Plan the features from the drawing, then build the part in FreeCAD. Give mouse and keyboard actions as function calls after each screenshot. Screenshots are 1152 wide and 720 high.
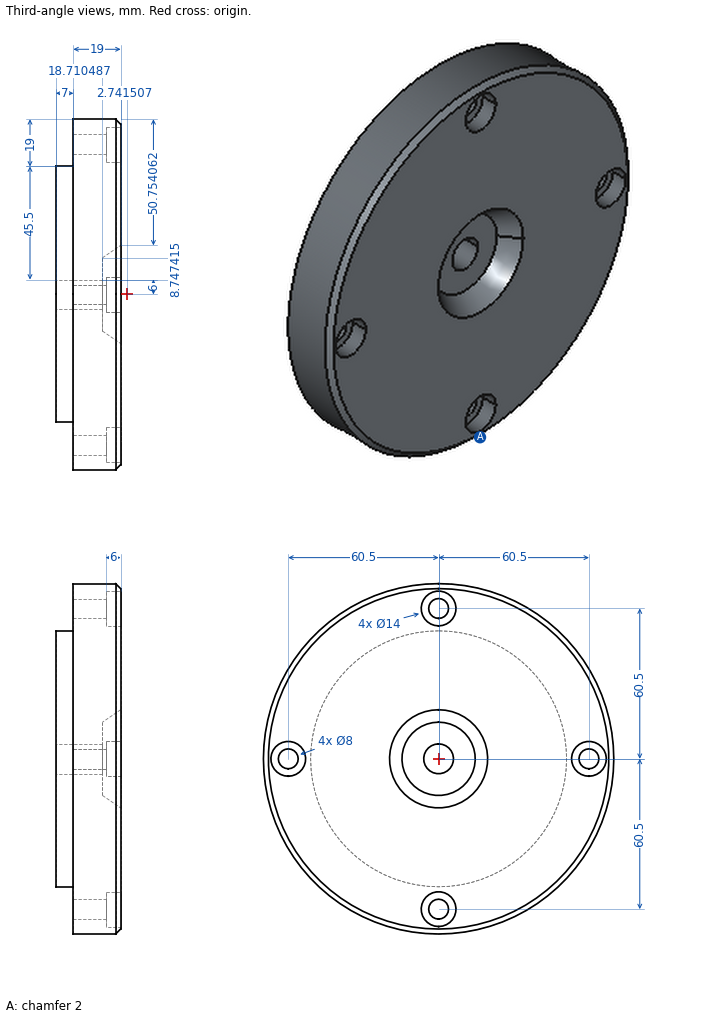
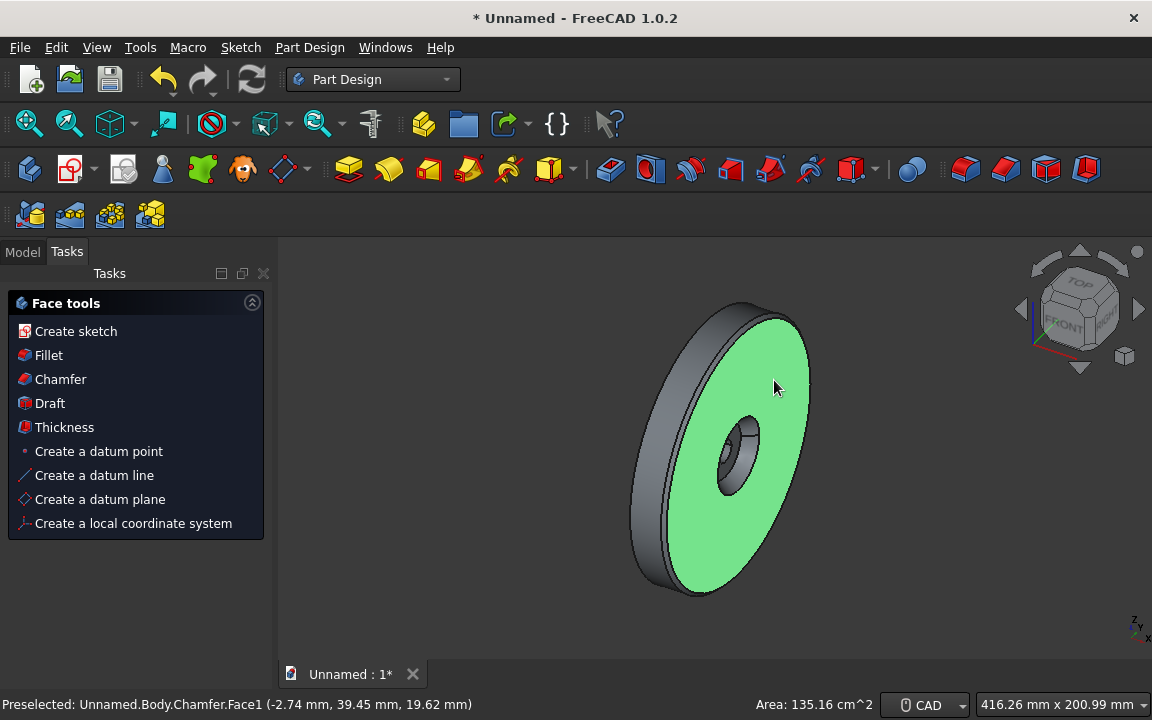
click(70, 170)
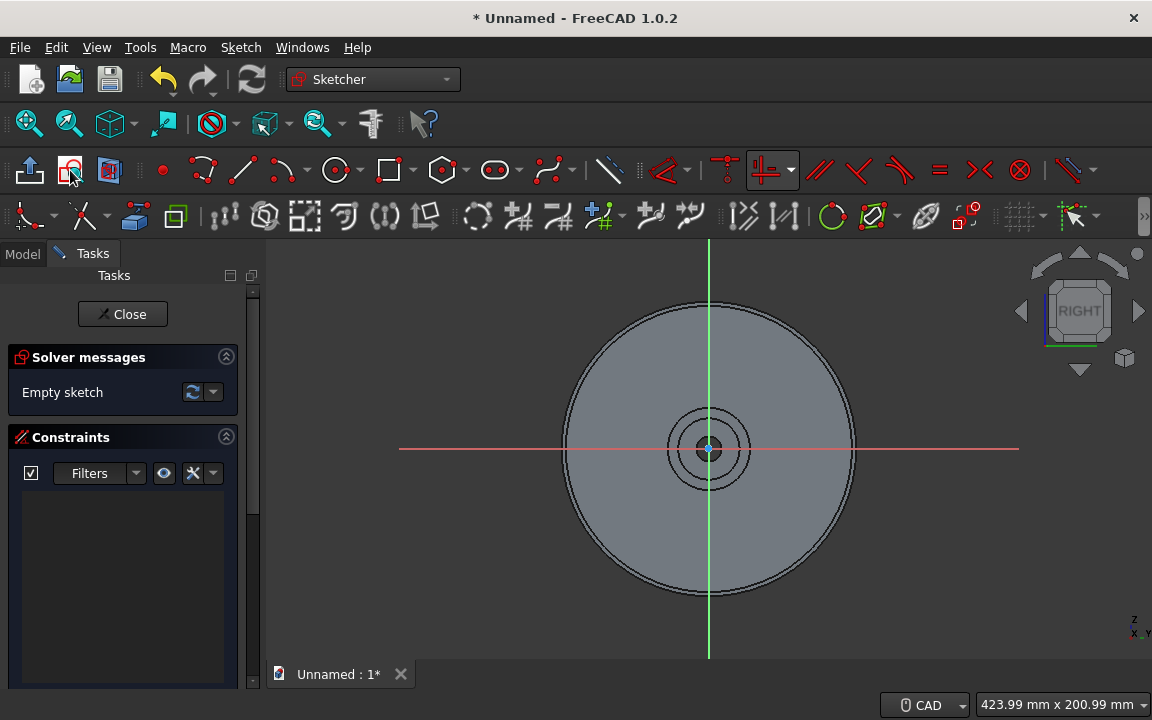
key(g)
key(c)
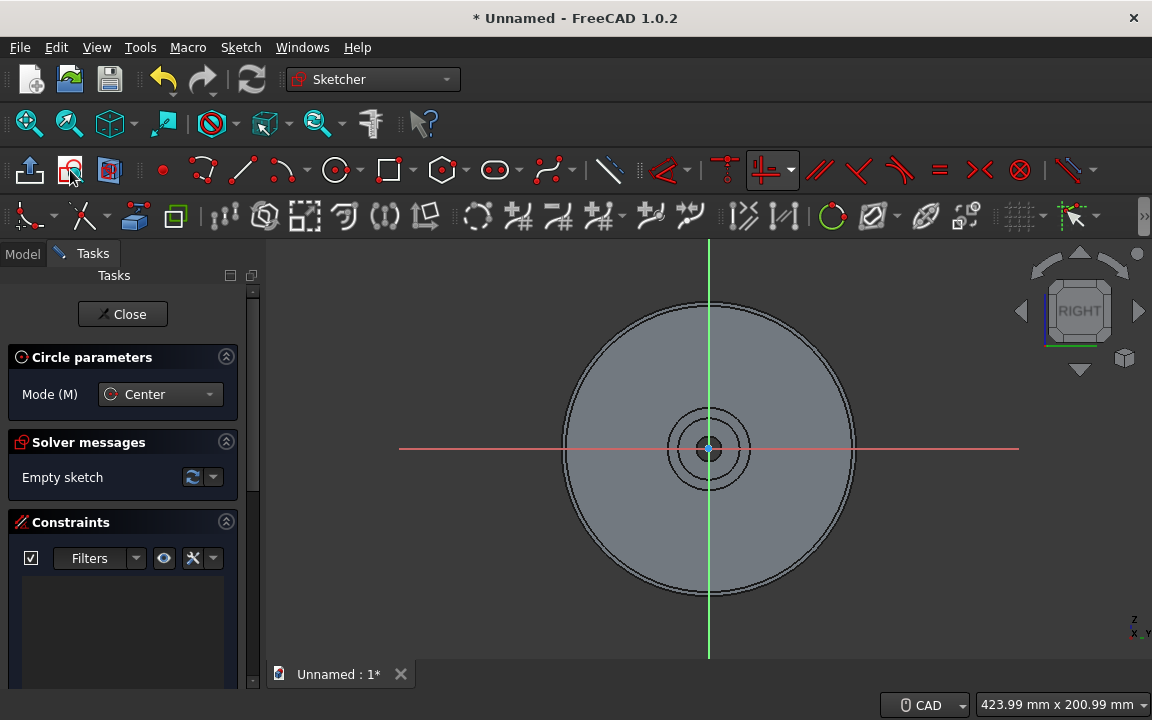
scroll(582, 449, up, 5)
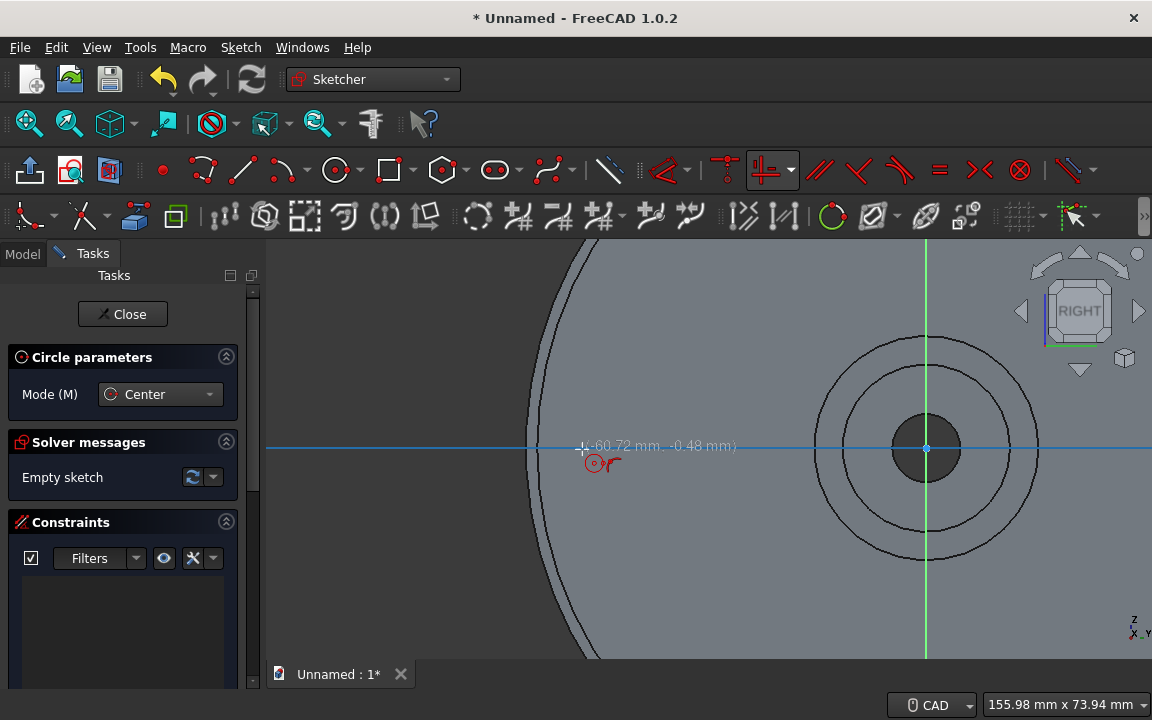
click(583, 448)
move(599, 432)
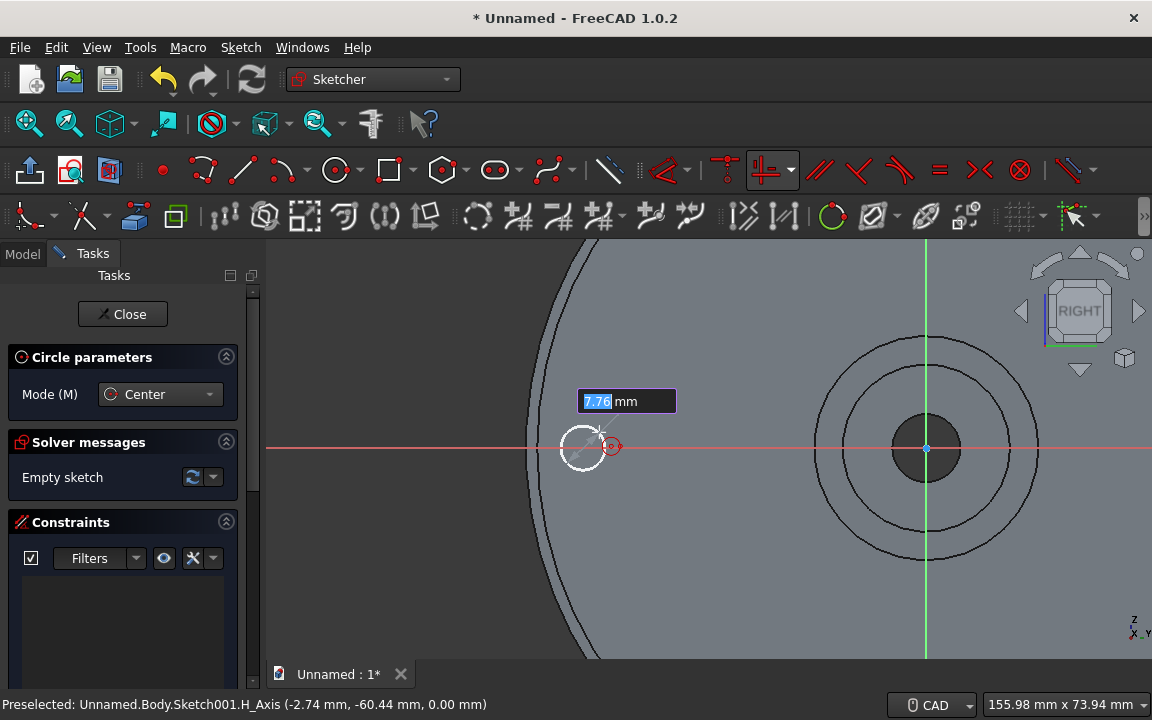
text(8)
key(Return)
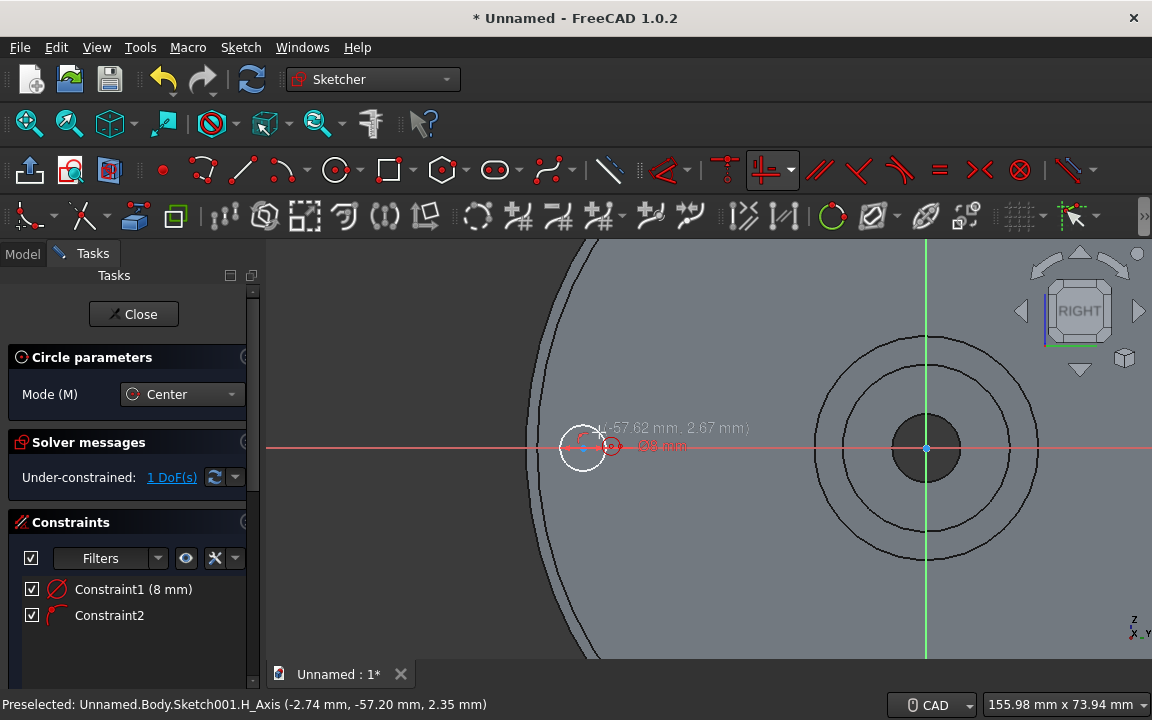
scroll(474, 450, down, 5)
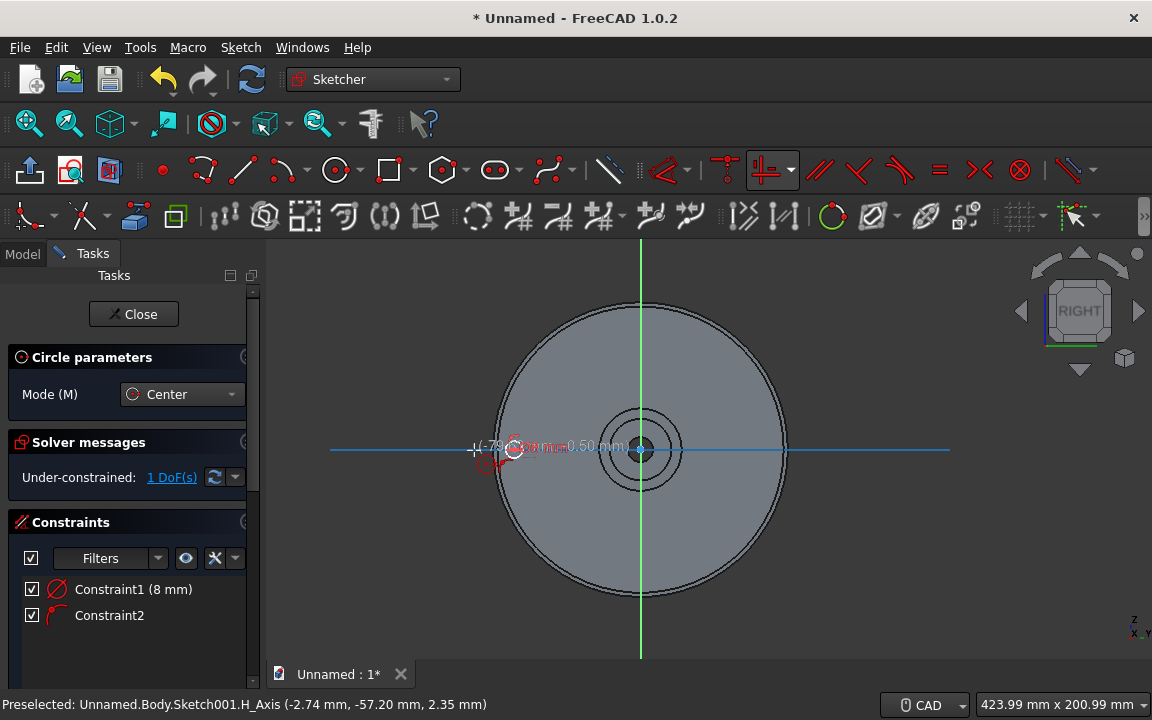
scroll(641, 323, up, 5)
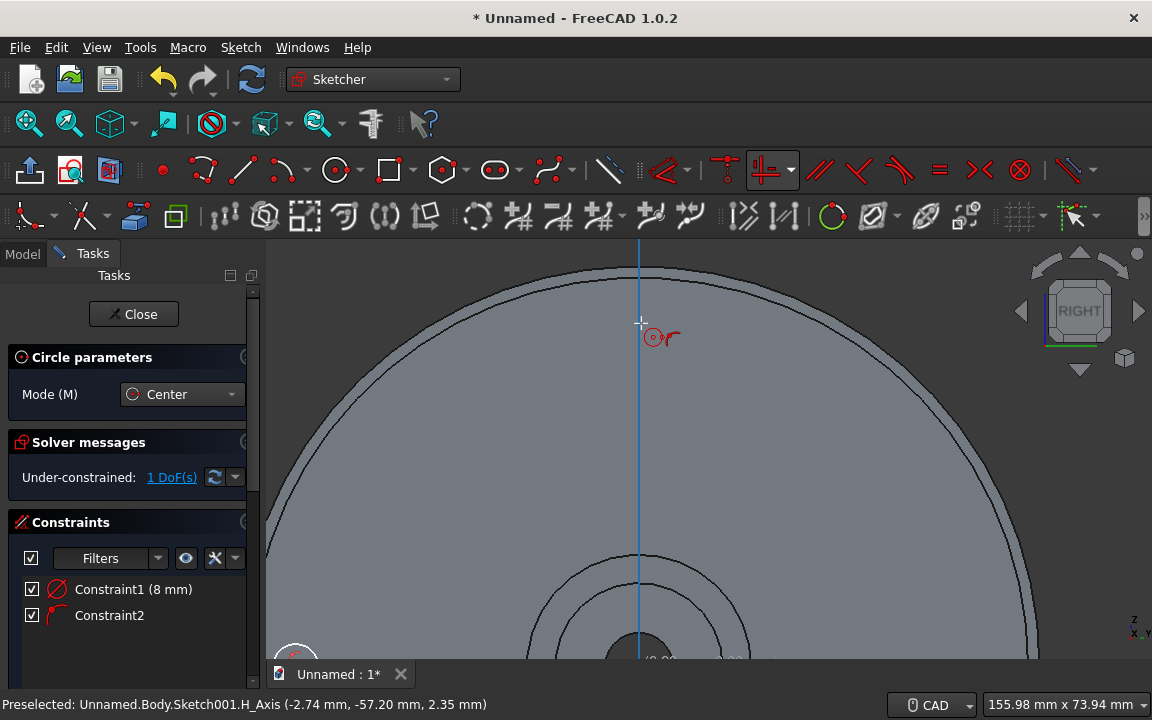
click(639, 323)
move(655, 307)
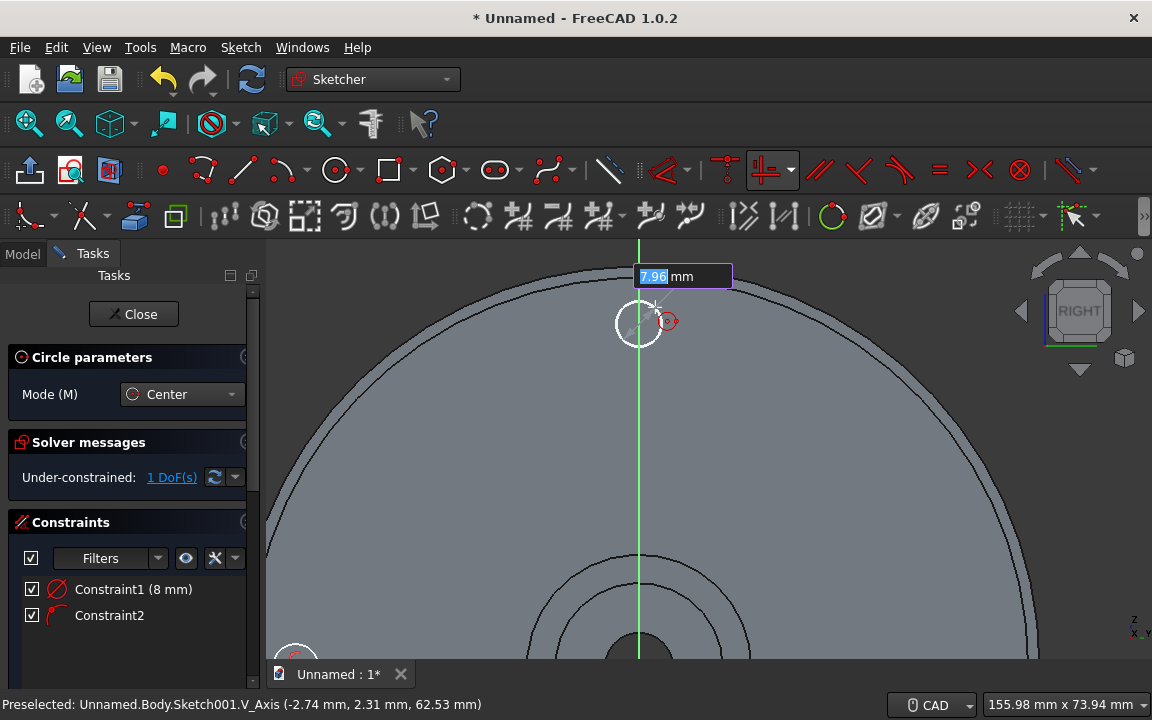
text(8)
key(Return)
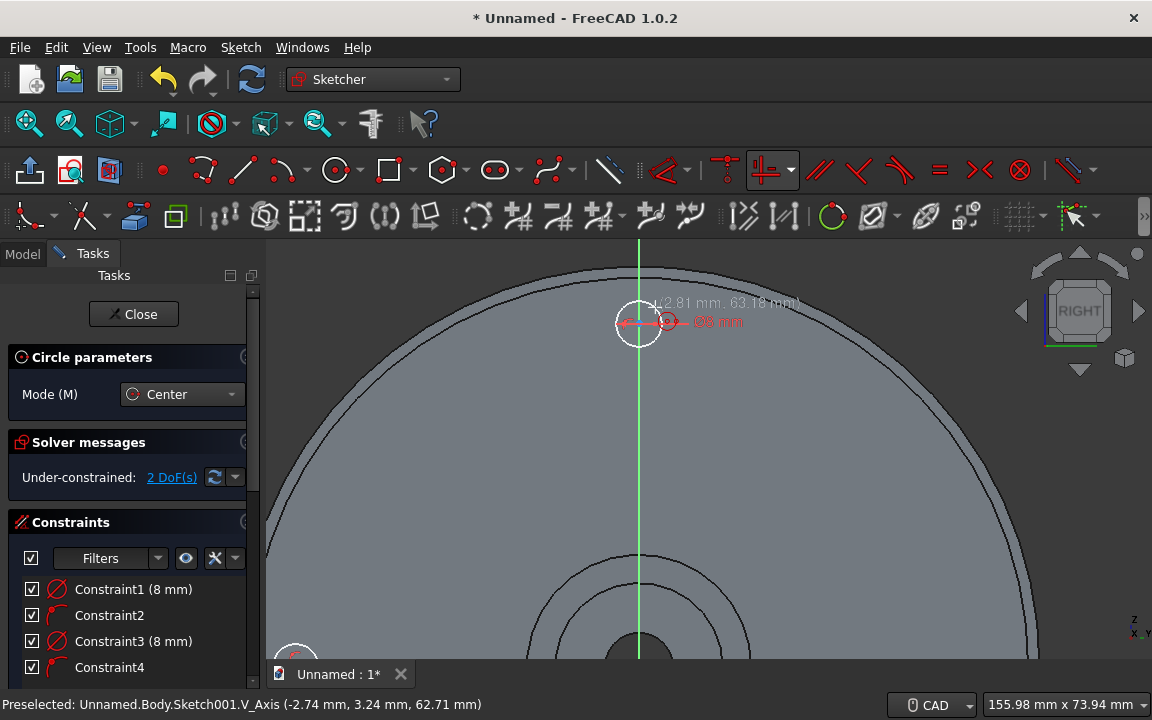
scroll(641, 322, down, 5)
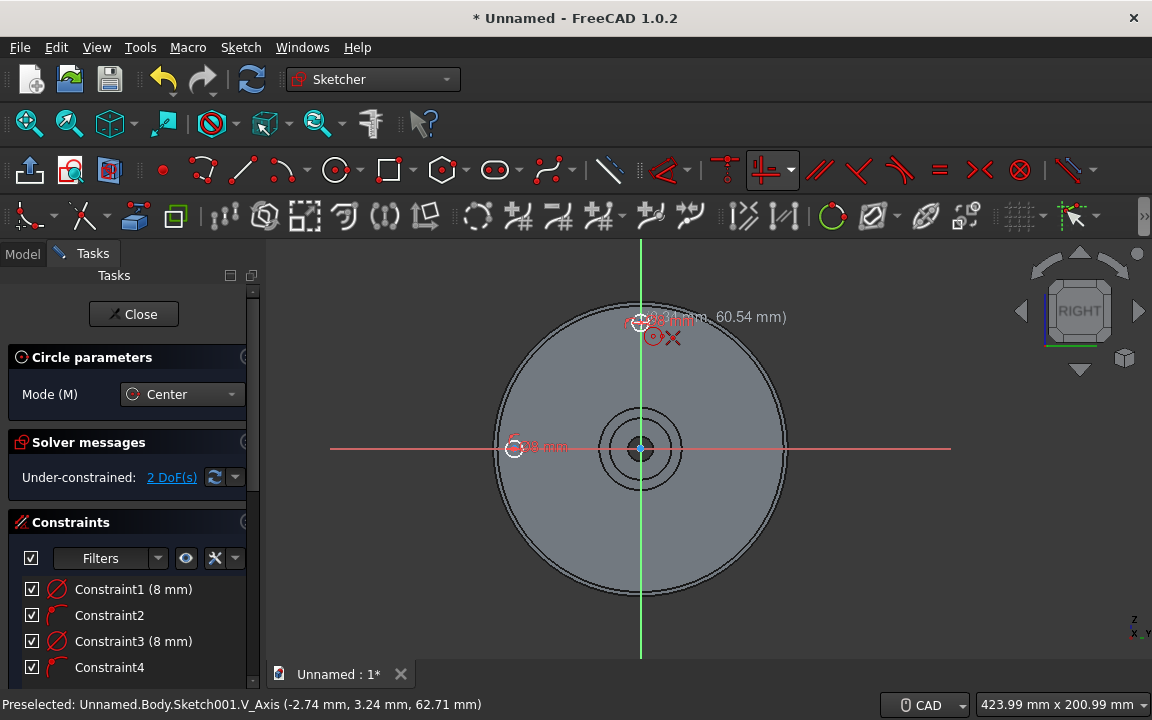
scroll(767, 449, up, 5)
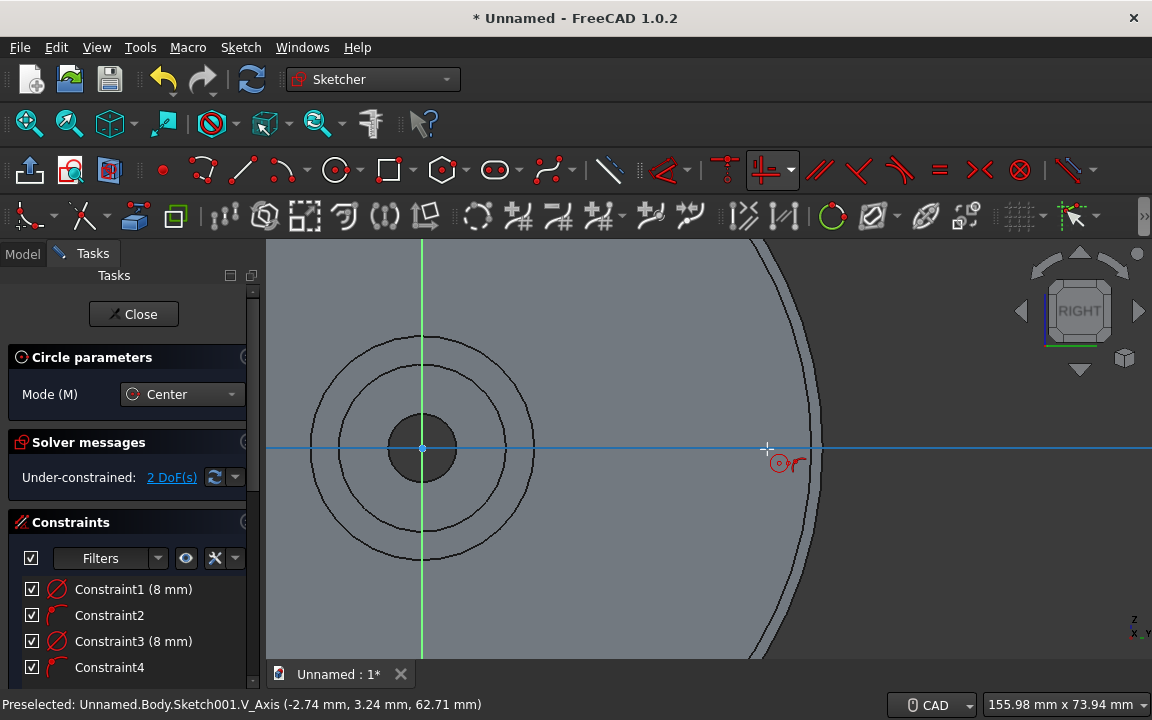
click(766, 448)
move(782, 432)